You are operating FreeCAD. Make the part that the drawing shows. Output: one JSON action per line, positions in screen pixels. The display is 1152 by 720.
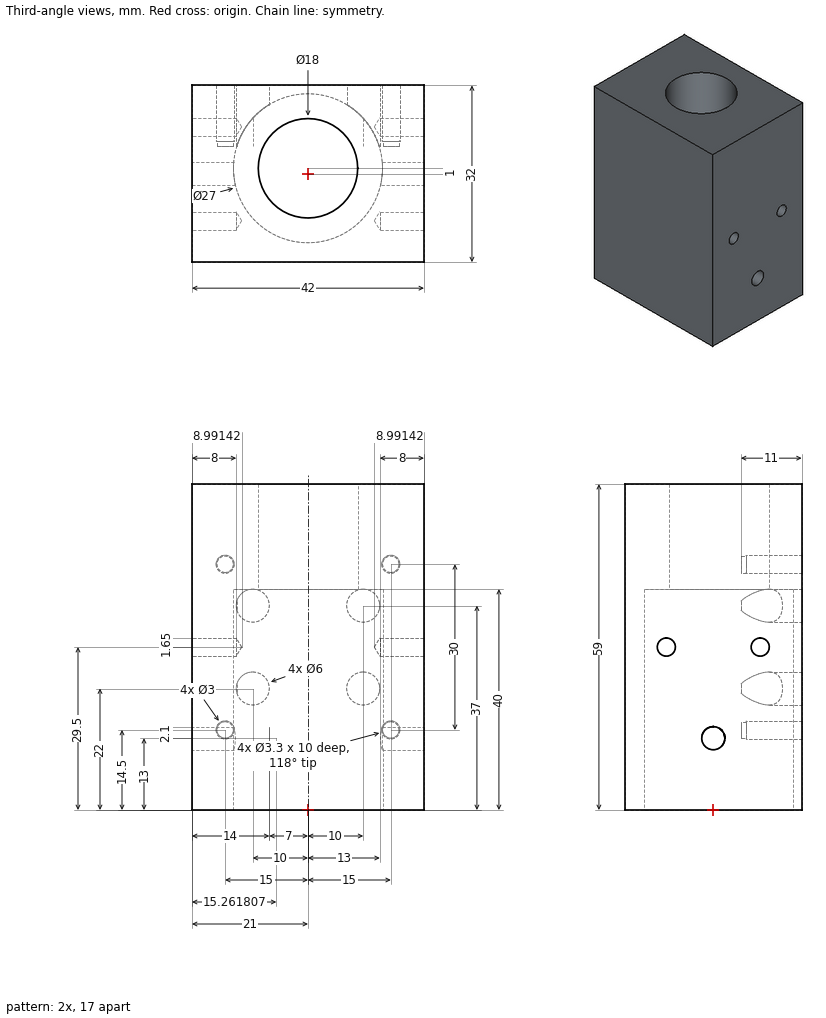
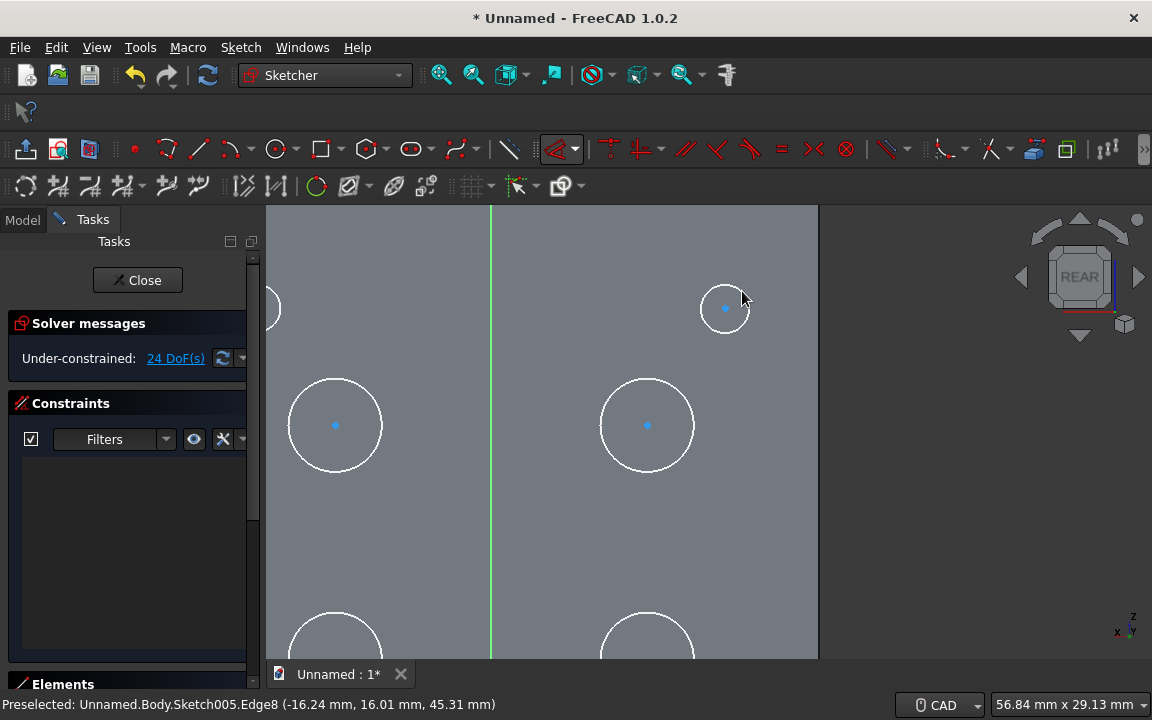
{"action": "left_click", "coordinate": [680, 626]}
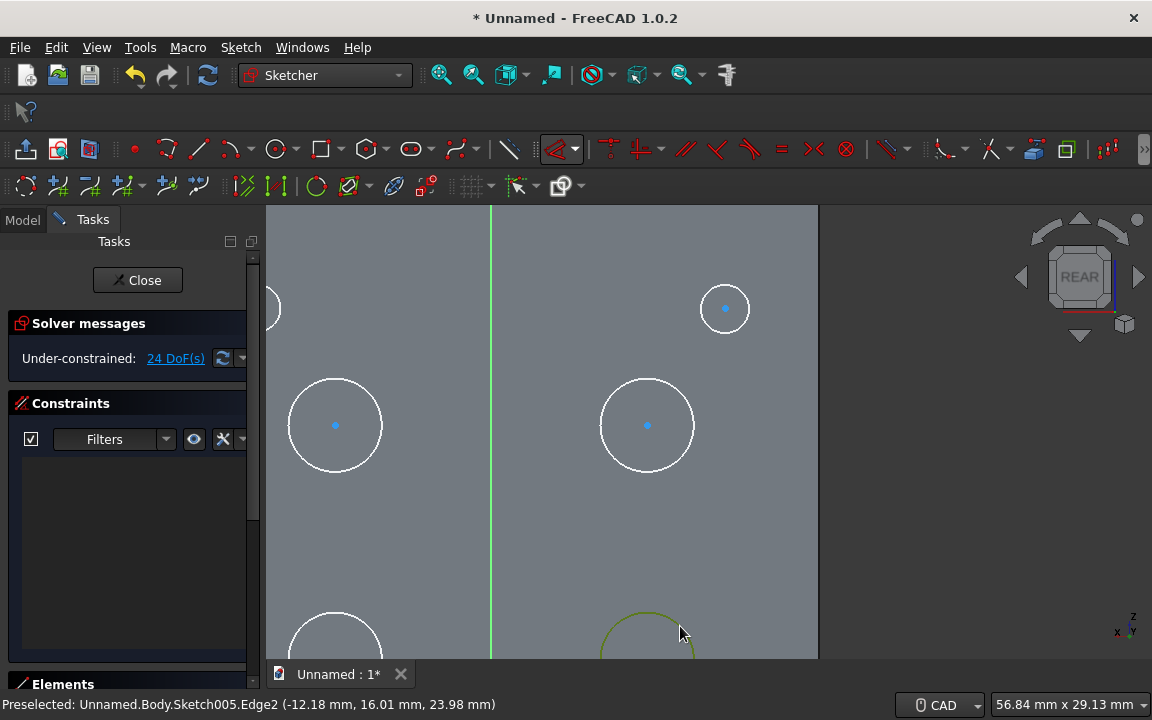
{"action": "left_click", "coordinate": [368, 626]}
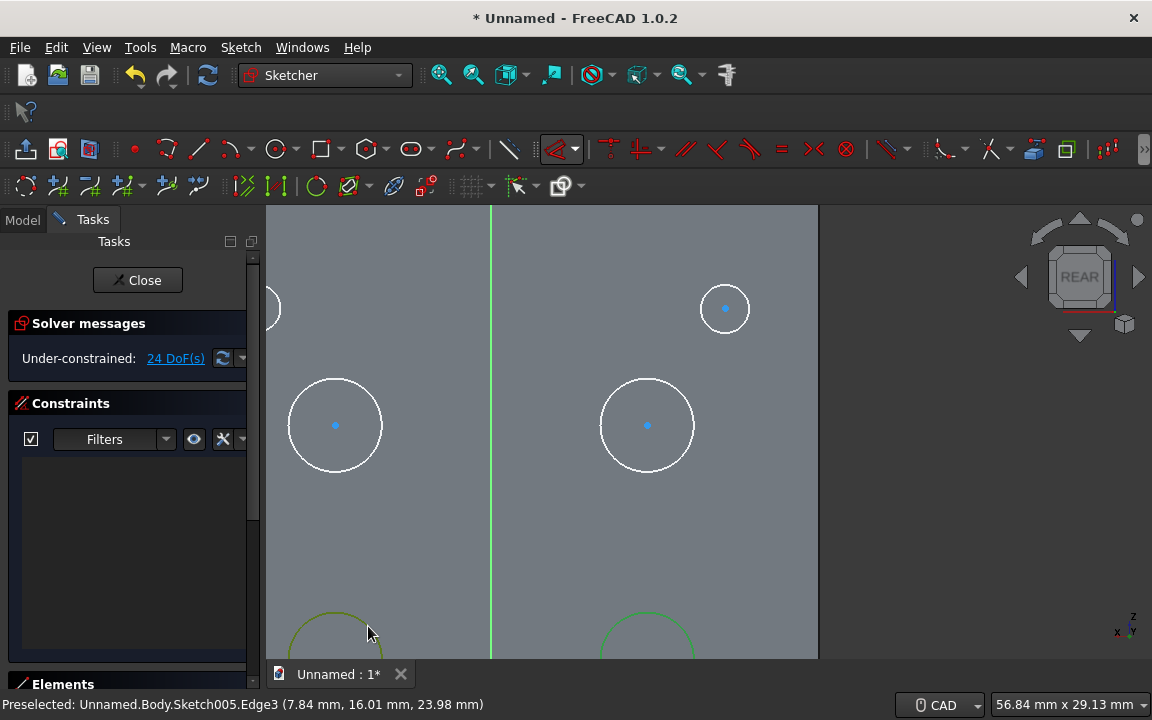
{"action": "left_click", "coordinate": [368, 392]}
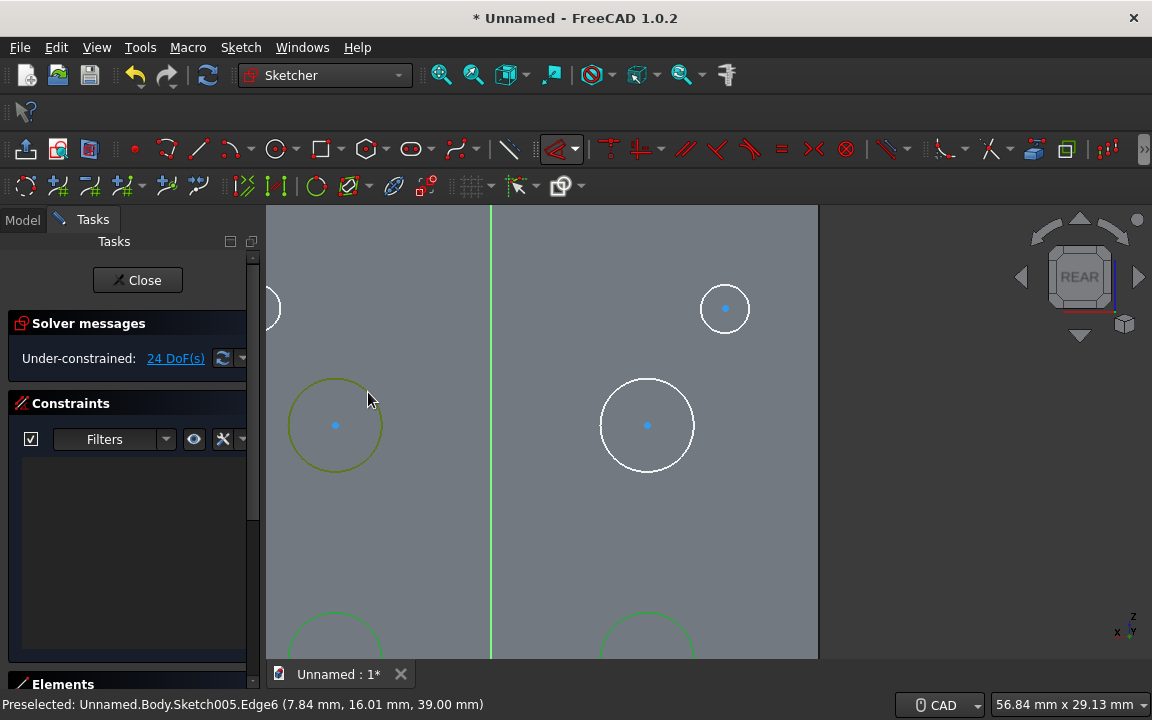
{"action": "left_click", "coordinate": [680, 392]}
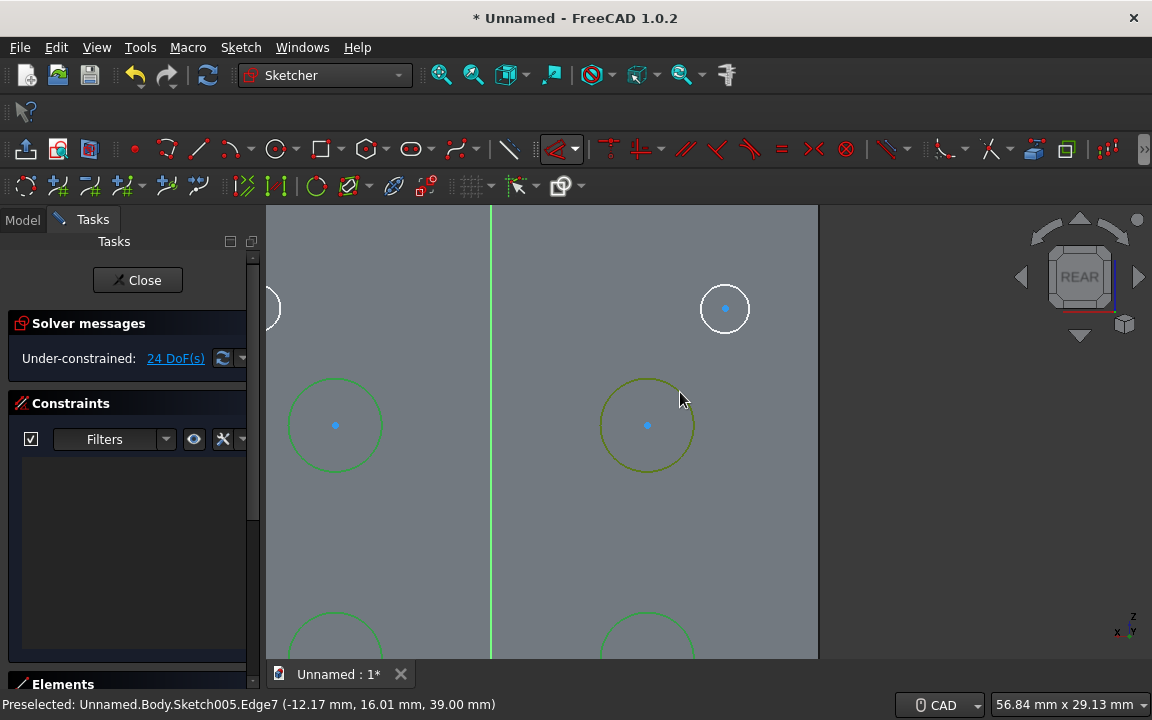
{"action": "key", "text": "e"}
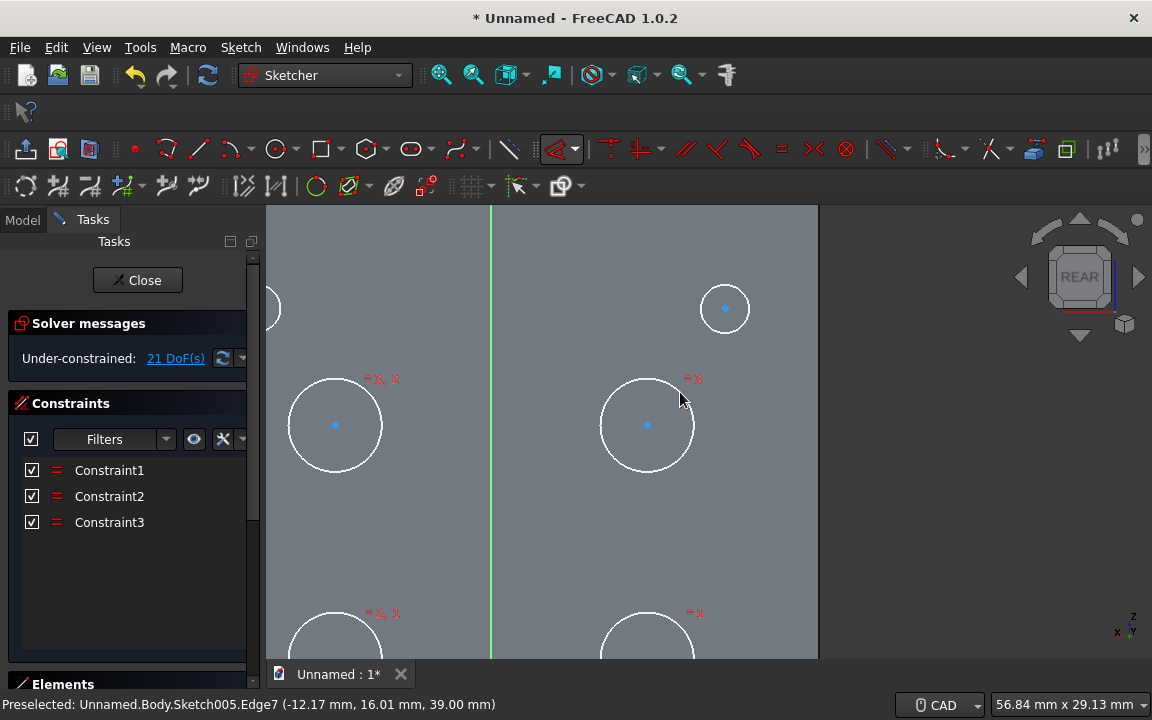
{"action": "scroll", "coordinate": [727, 309], "scroll_direction": "down", "scroll_amount": 5}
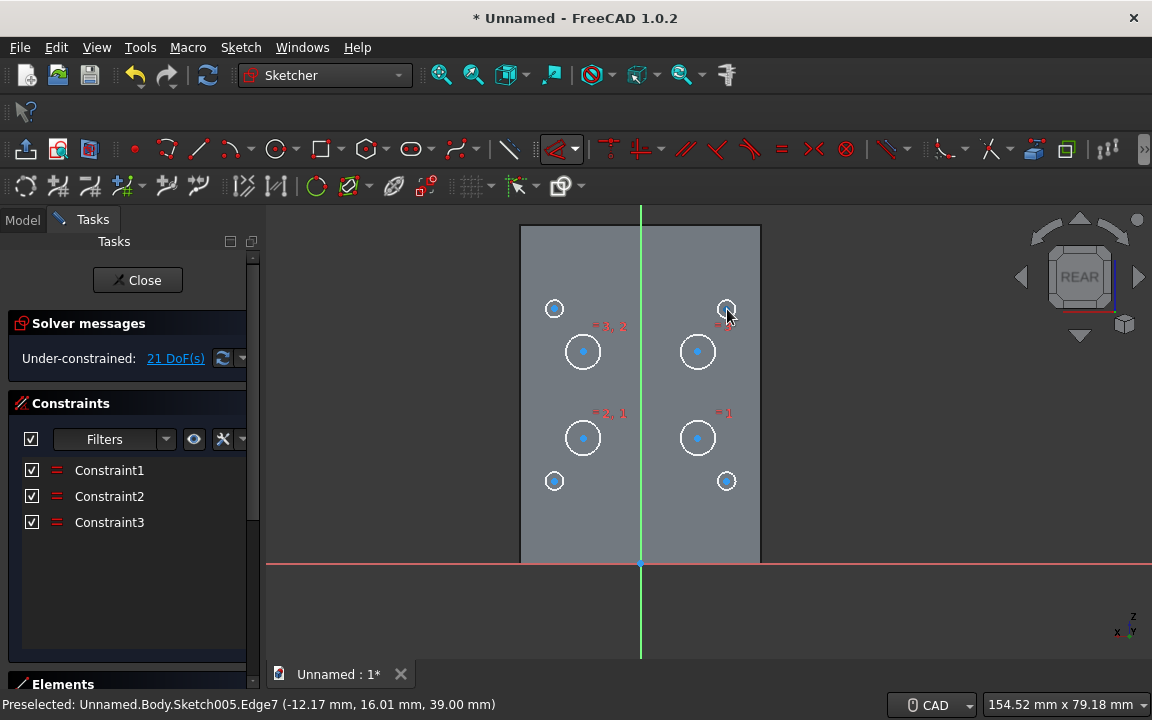
{"action": "scroll", "coordinate": [733, 475], "scroll_direction": "up", "scroll_amount": 3}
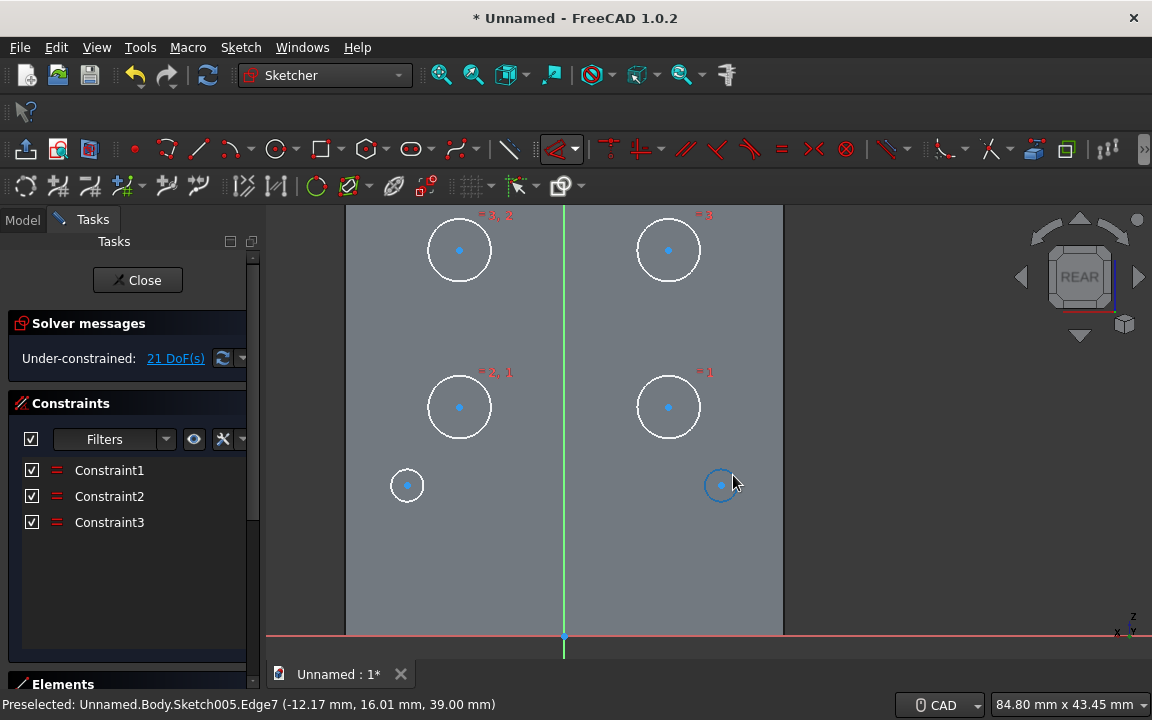
{"action": "left_click", "coordinate": [732, 474]}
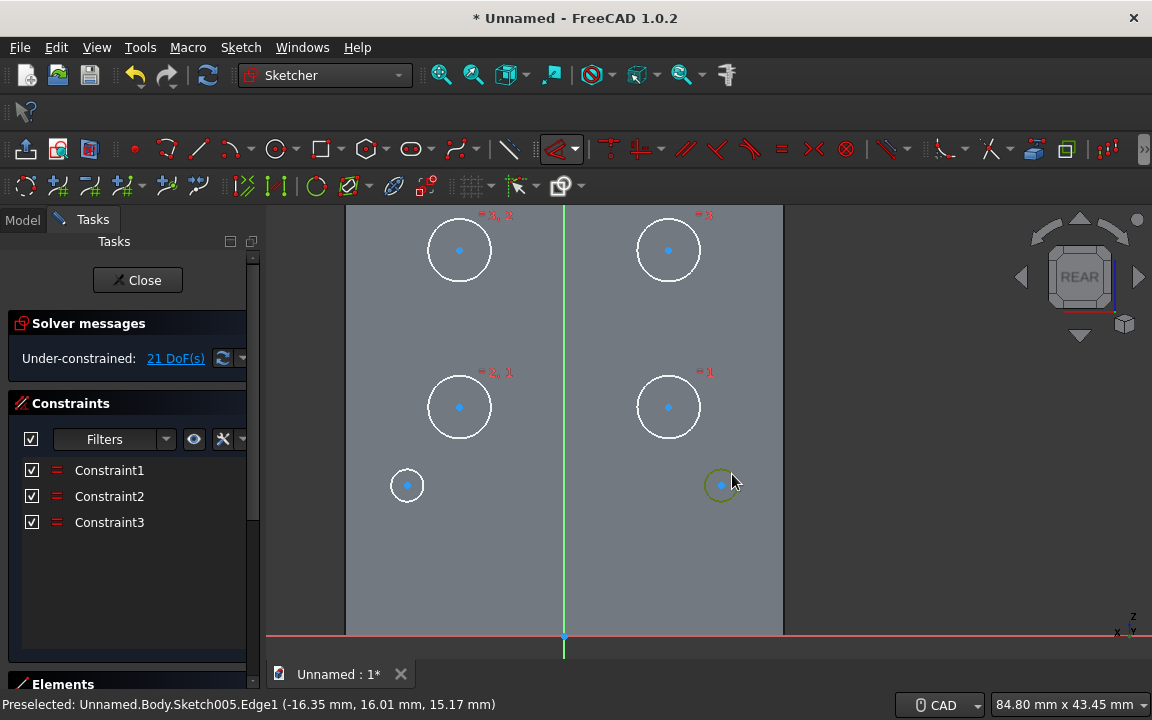
{"action": "left_click", "coordinate": [419, 474]}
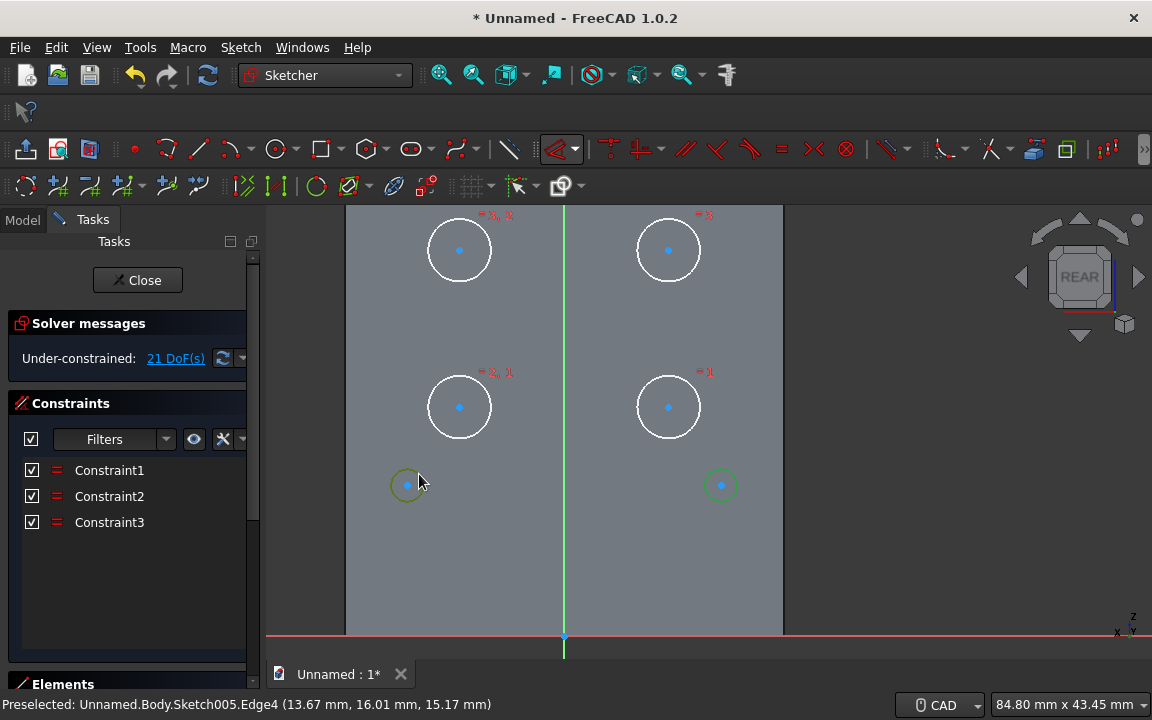
{"action": "scroll", "coordinate": [733, 476], "scroll_direction": "down", "scroll_amount": 3}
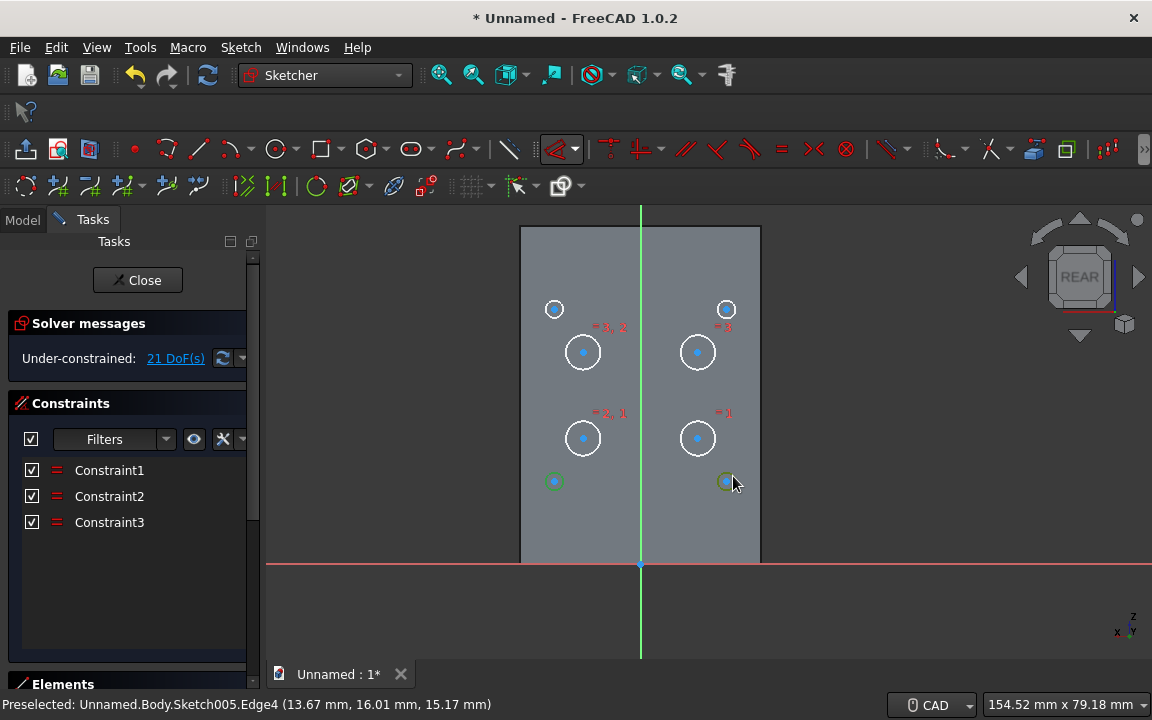
{"action": "scroll", "coordinate": [561, 303], "scroll_direction": "up", "scroll_amount": 3}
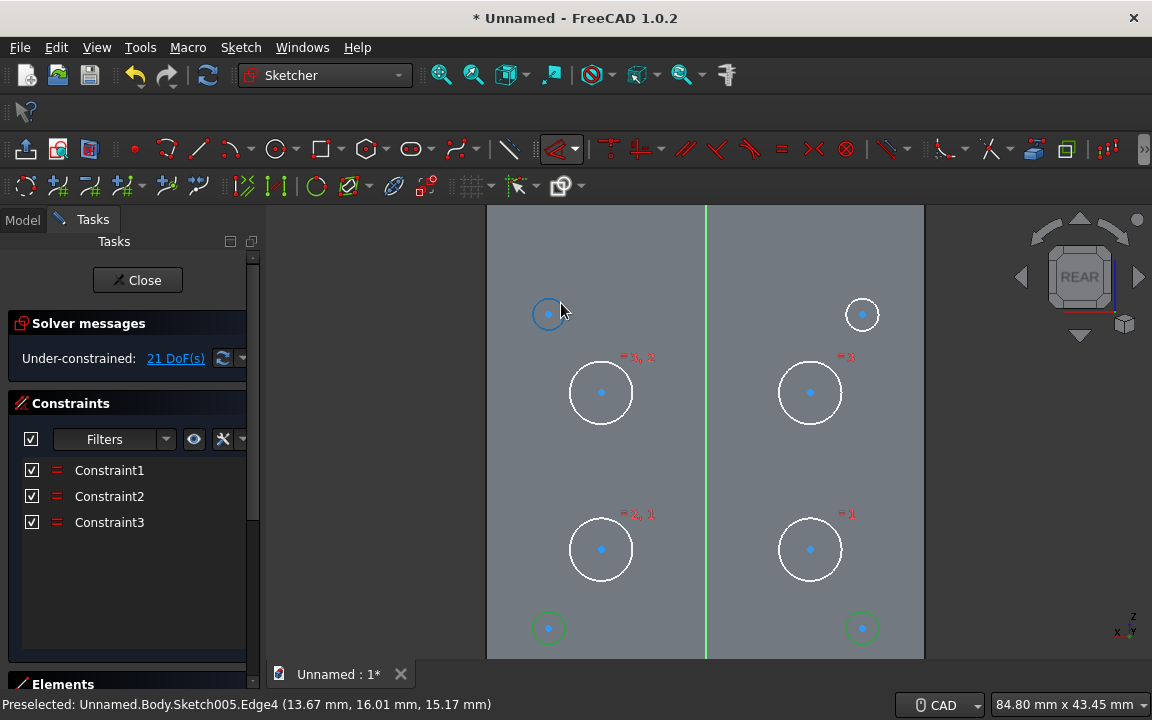
{"action": "left_click", "coordinate": [560, 303]}